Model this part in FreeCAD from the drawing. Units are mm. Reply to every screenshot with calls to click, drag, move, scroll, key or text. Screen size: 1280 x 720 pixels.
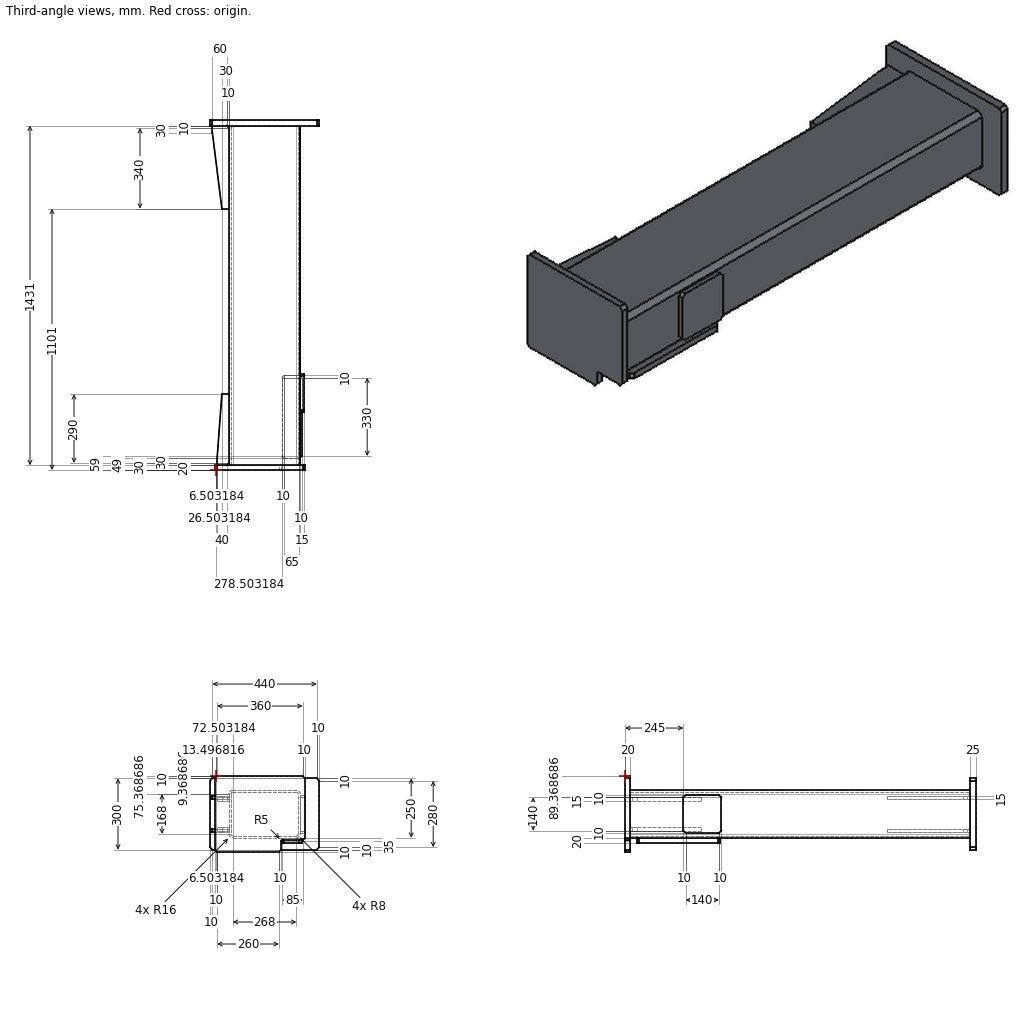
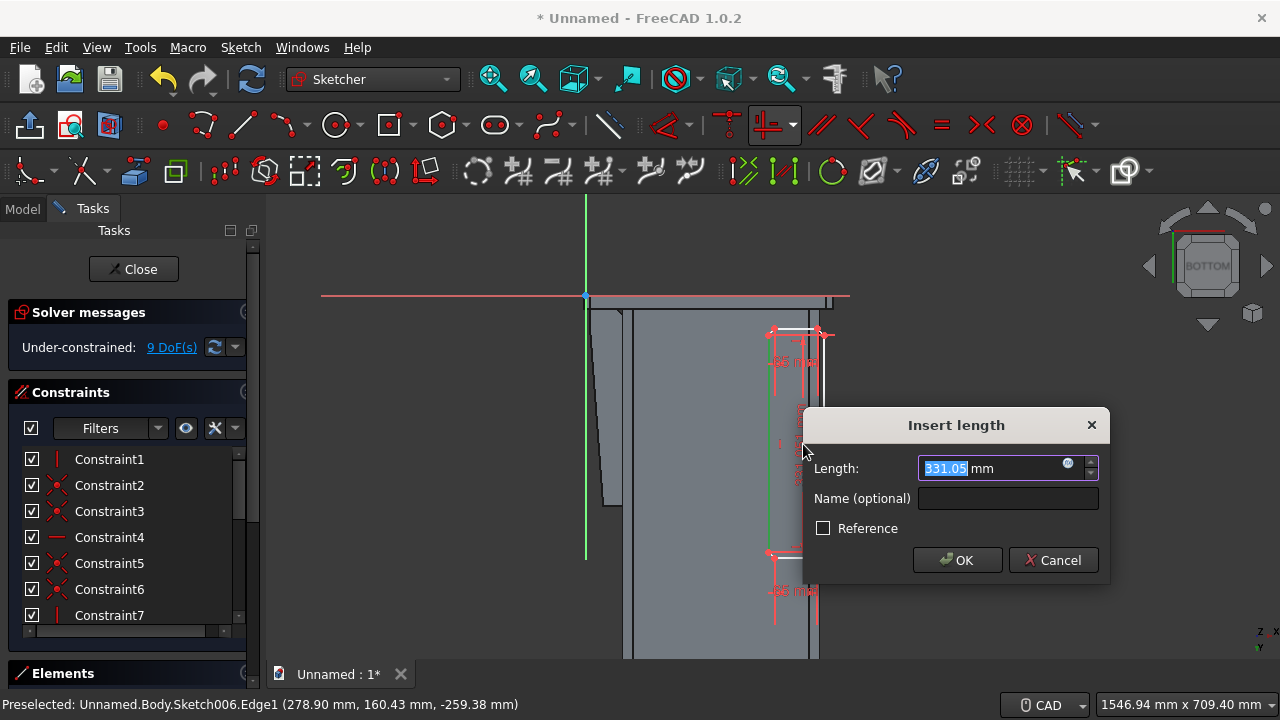
text(330)
key(Return)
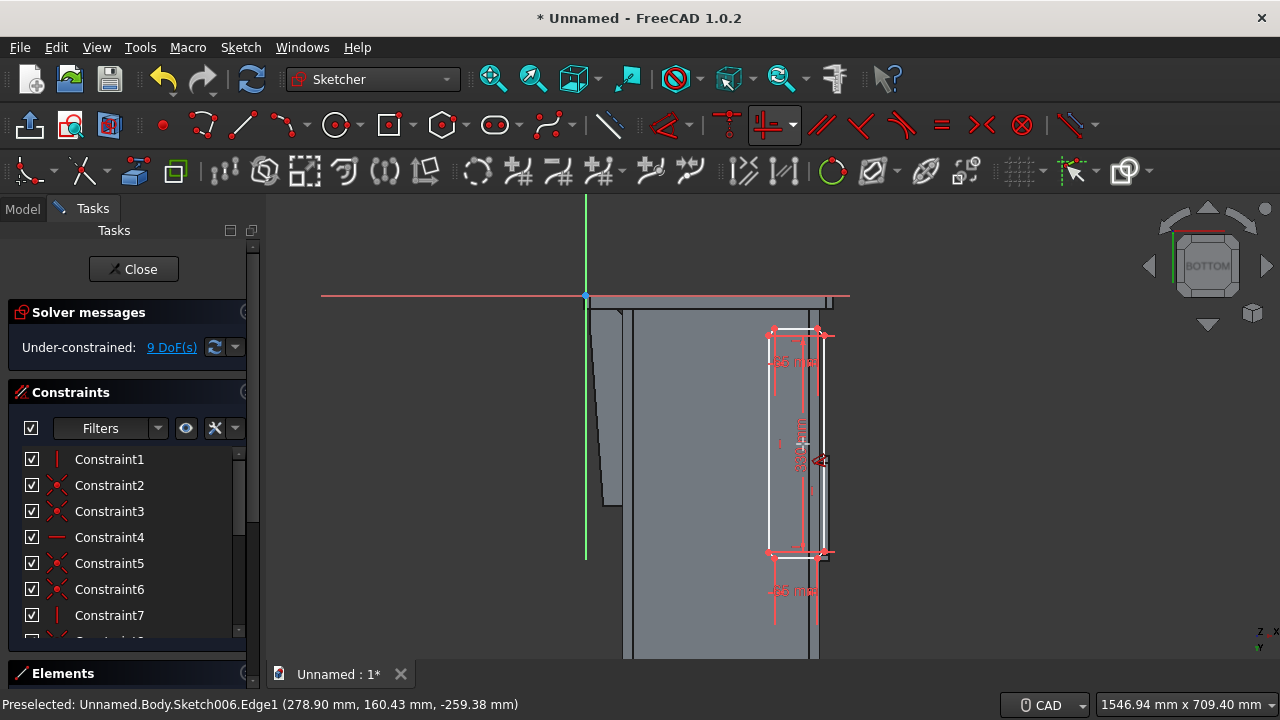
click(824, 487)
click(858, 394)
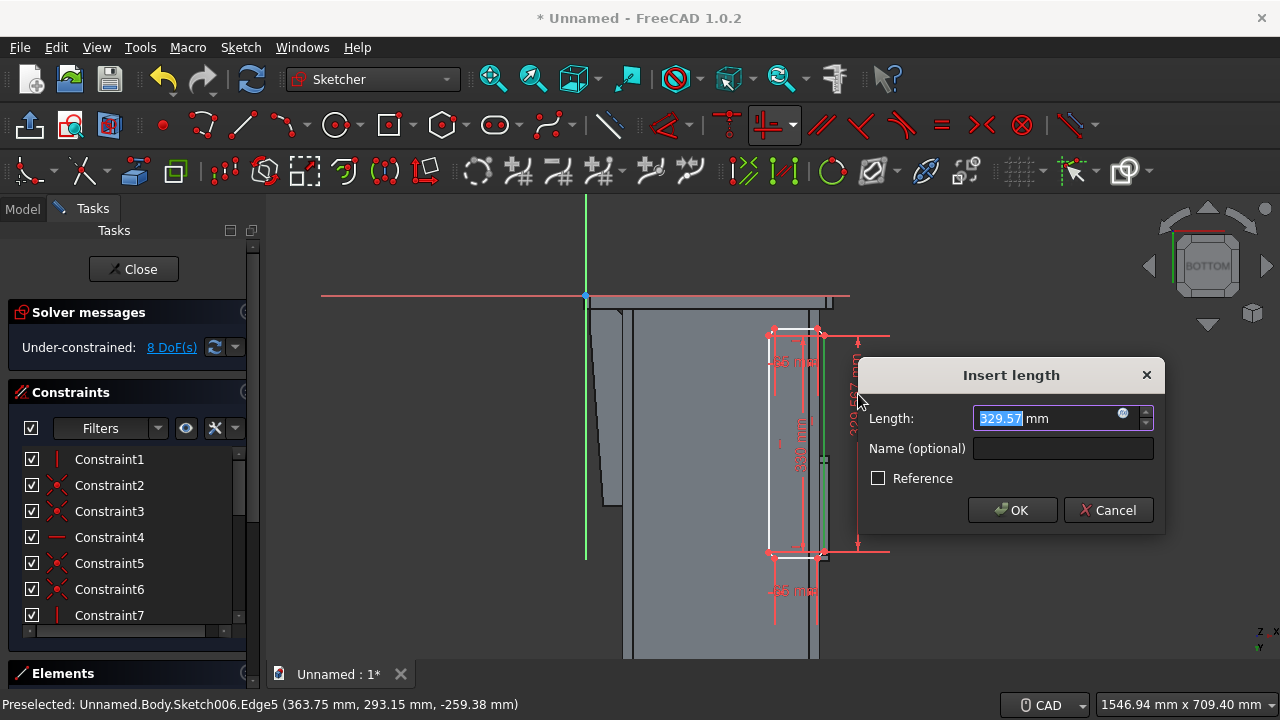
text(330)
key(Return)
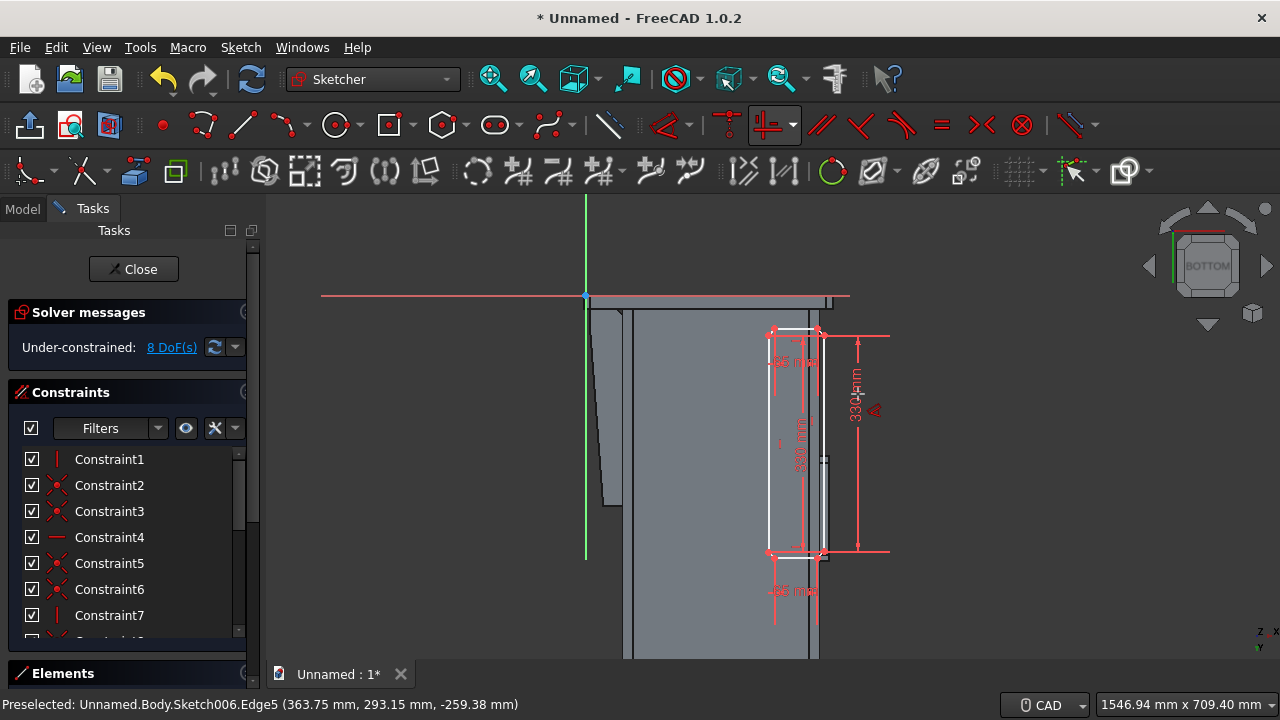
scroll(769, 336, up, 2)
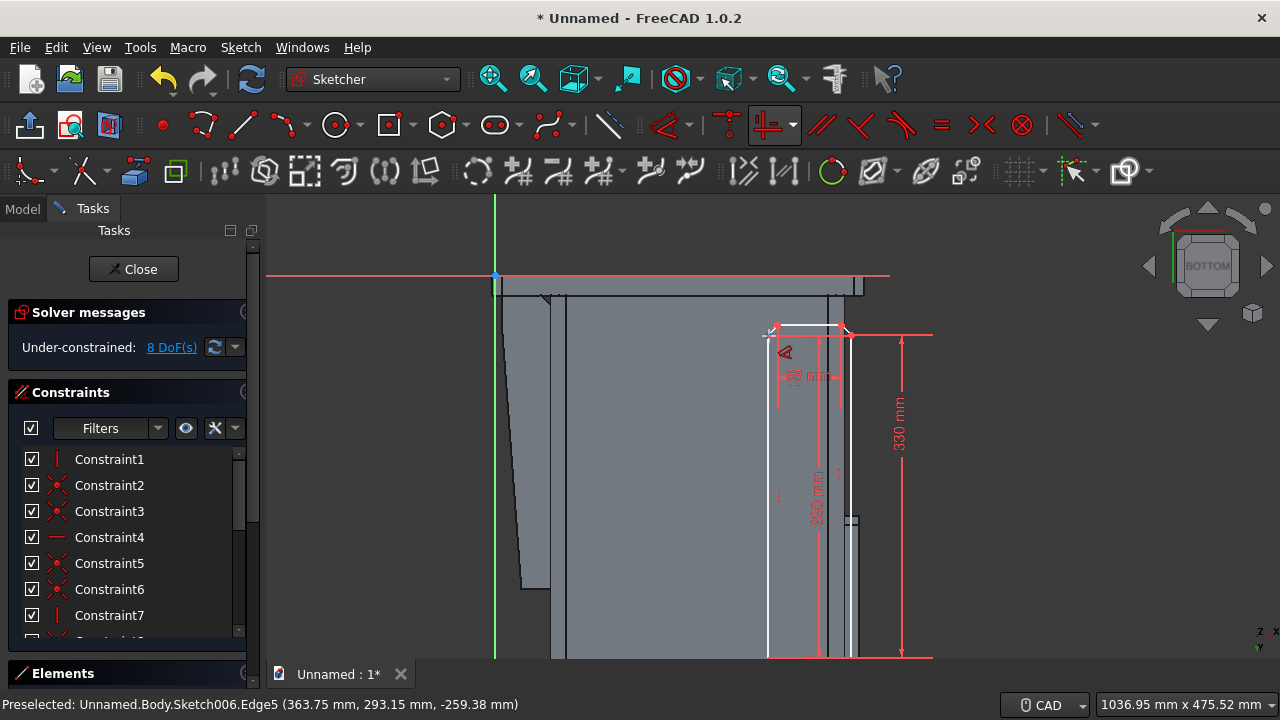
click(768, 335)
click(461, 306)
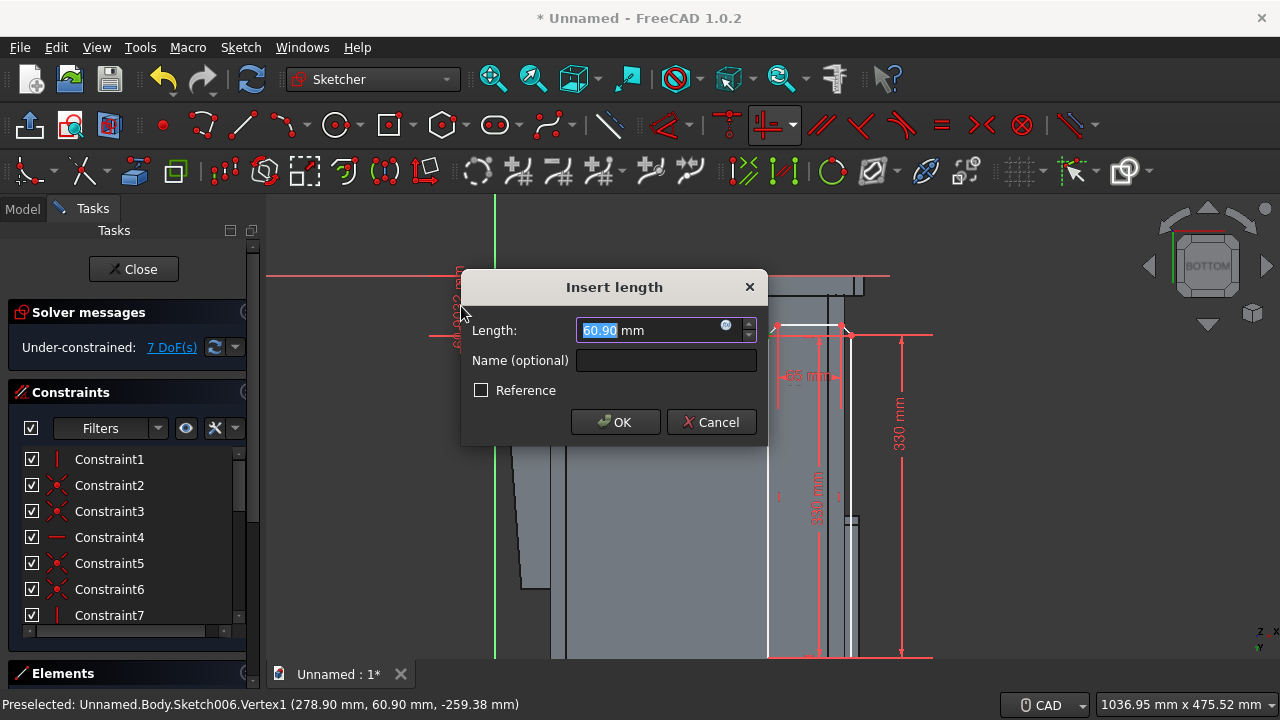
text(59)
key(Return)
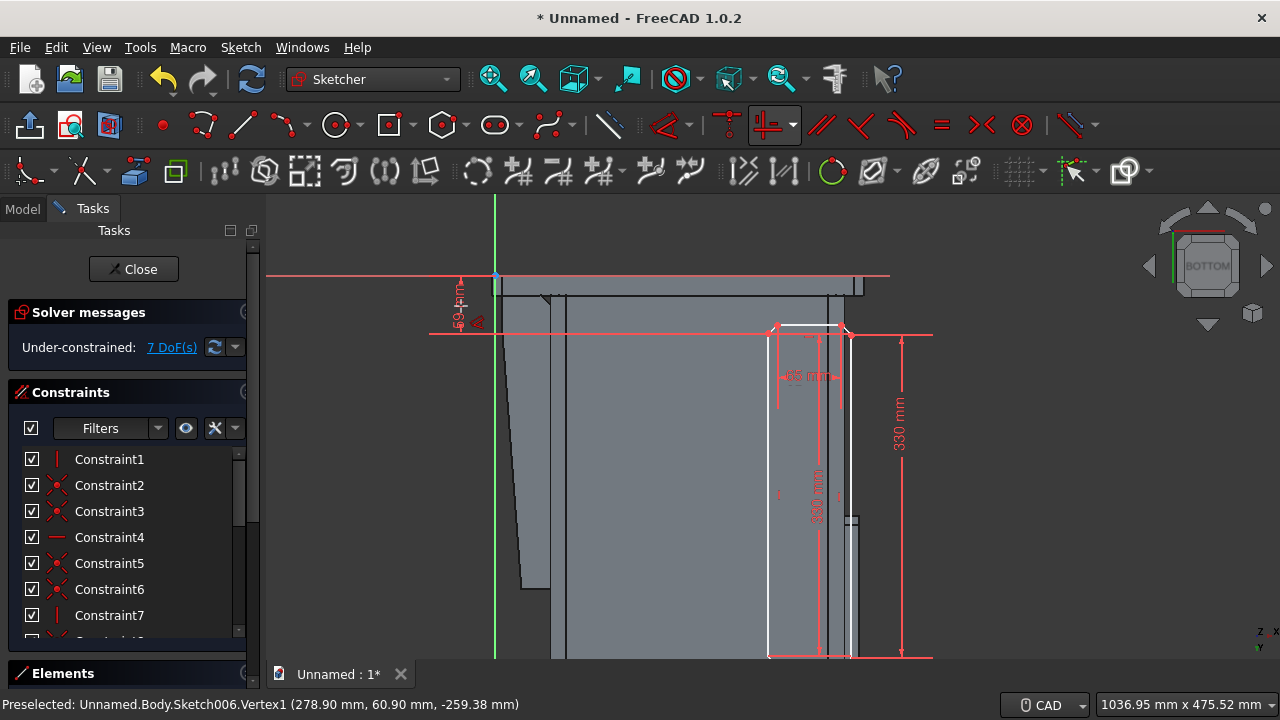
click(851, 335)
click(885, 306)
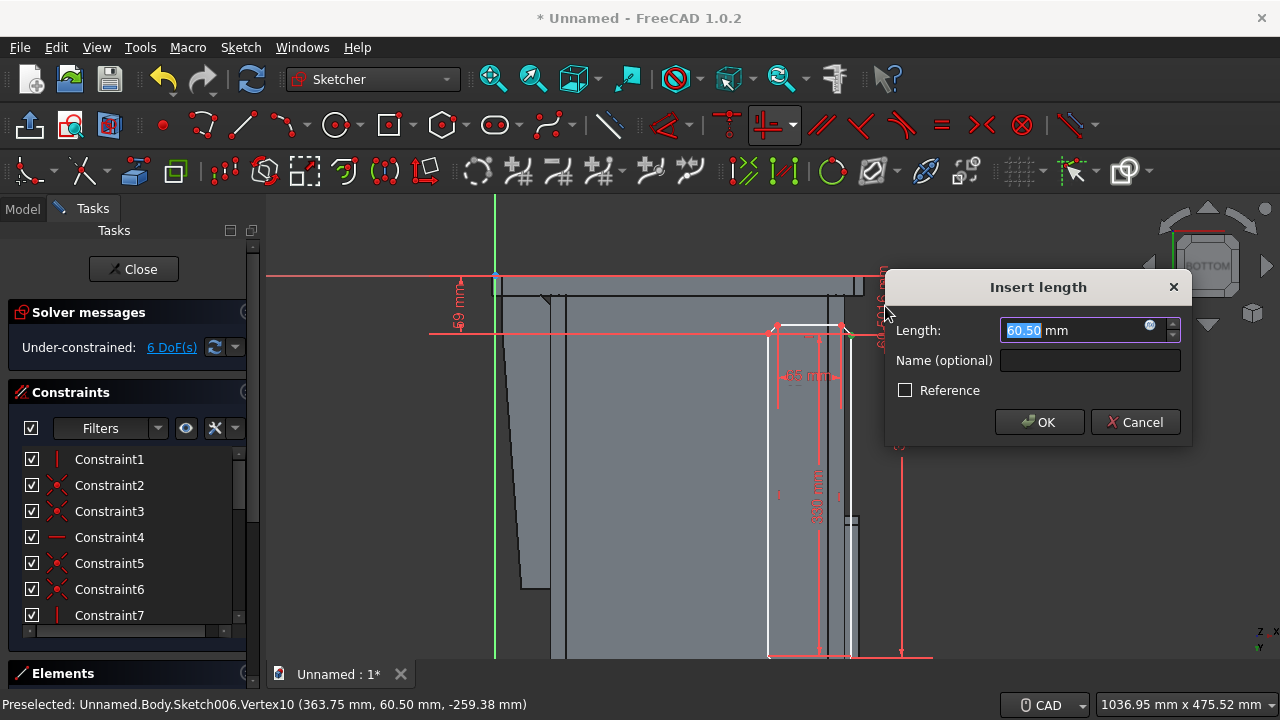
text(59)
key(Return)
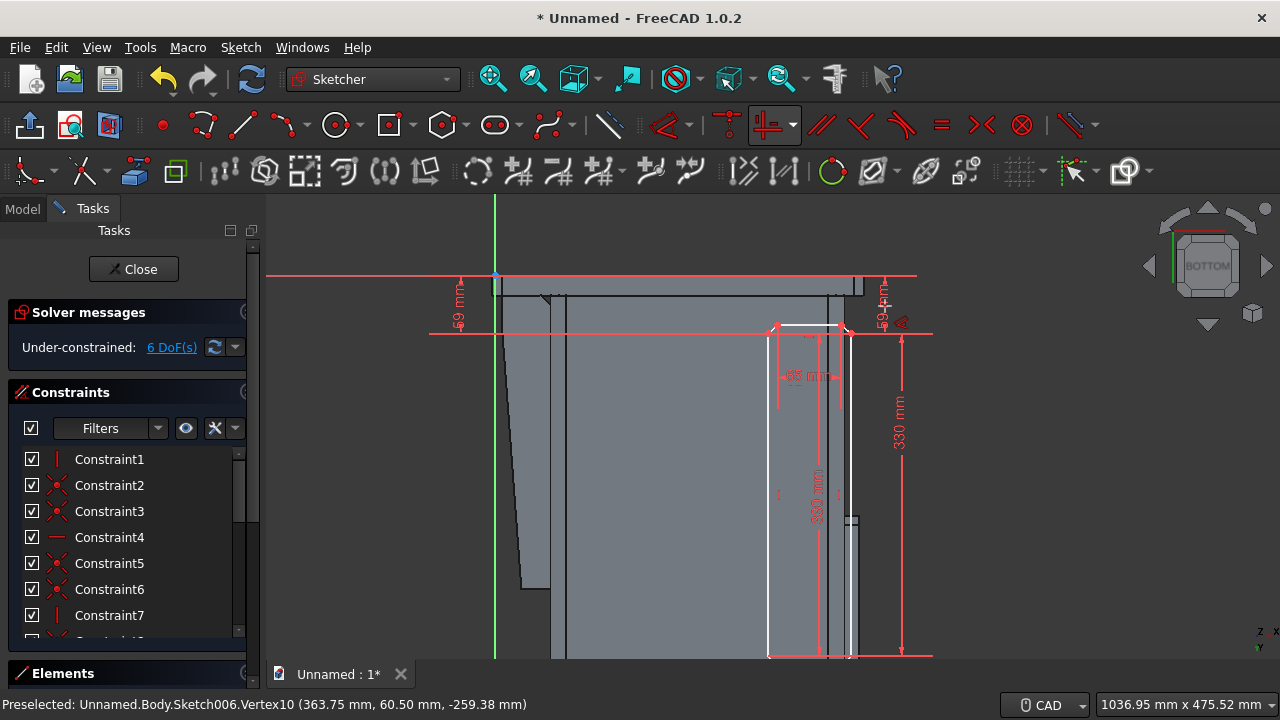
click(841, 325)
click(389, 301)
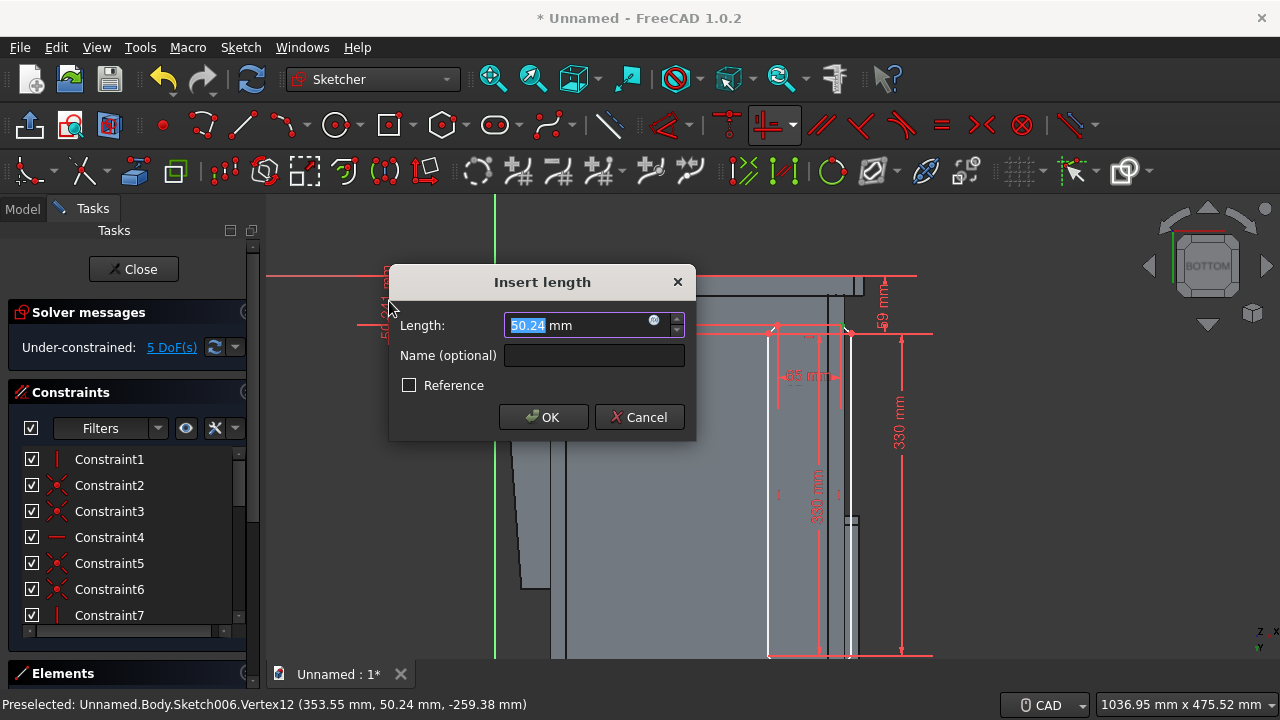
text(49)
key(Return)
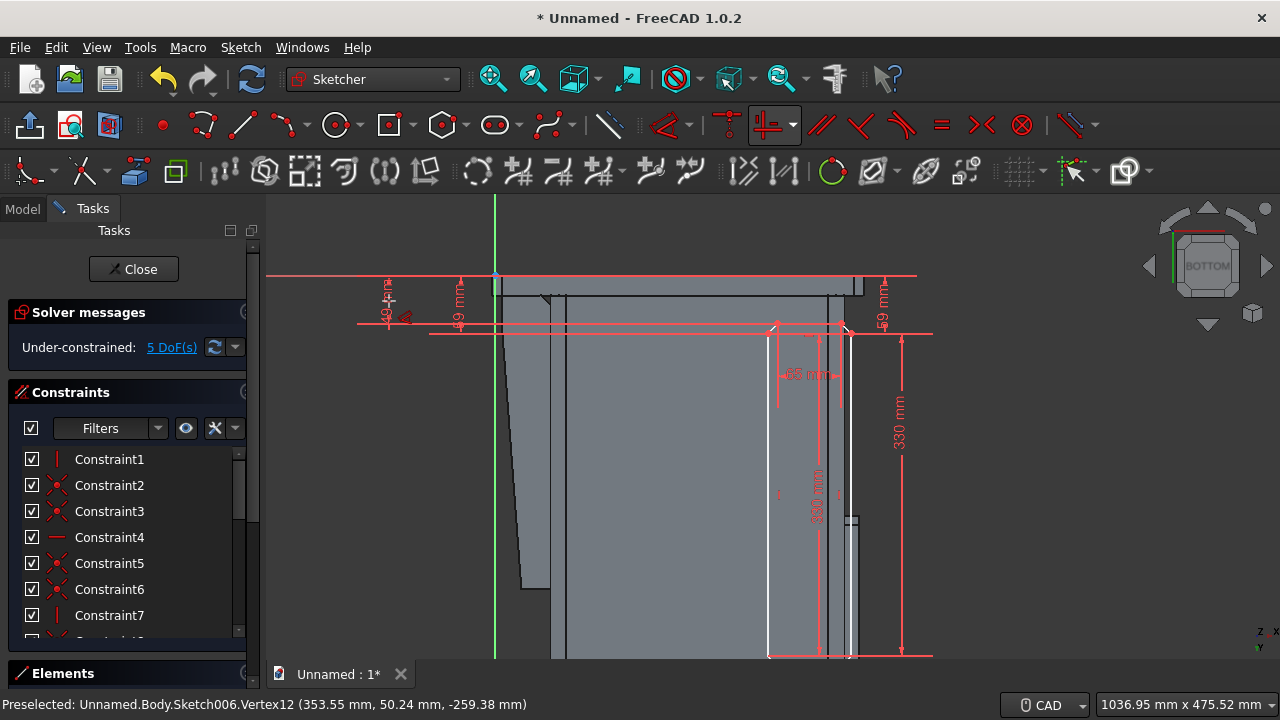
scroll(768, 336, down, 2)